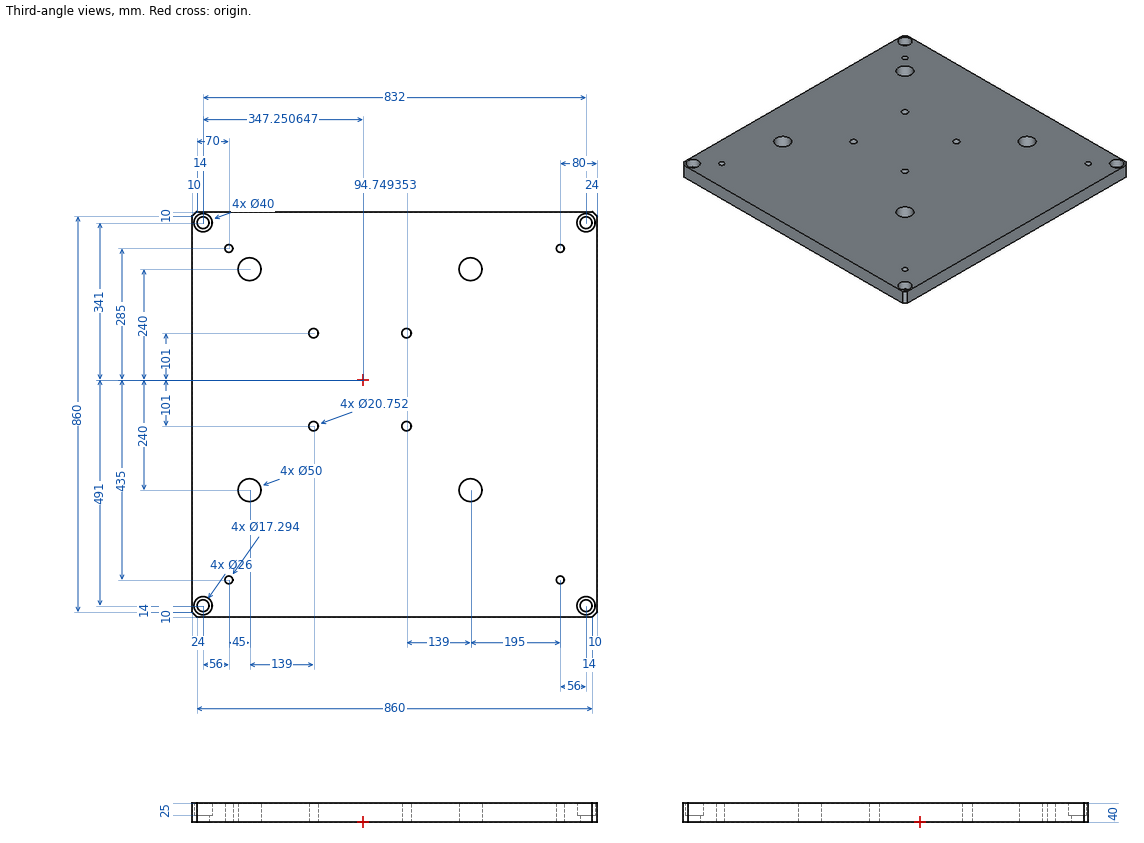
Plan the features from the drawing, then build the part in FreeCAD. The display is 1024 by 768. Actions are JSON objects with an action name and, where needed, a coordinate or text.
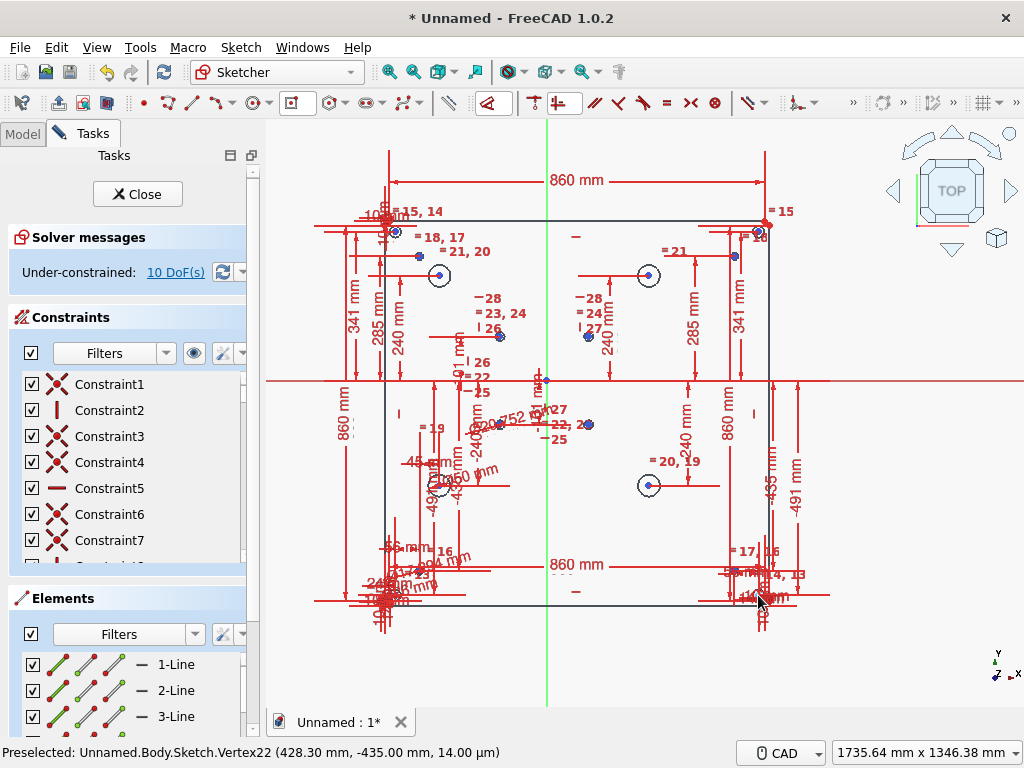
{"action": "scroll", "coordinate": [440, 276], "scroll_direction": "up", "scroll_amount": 4}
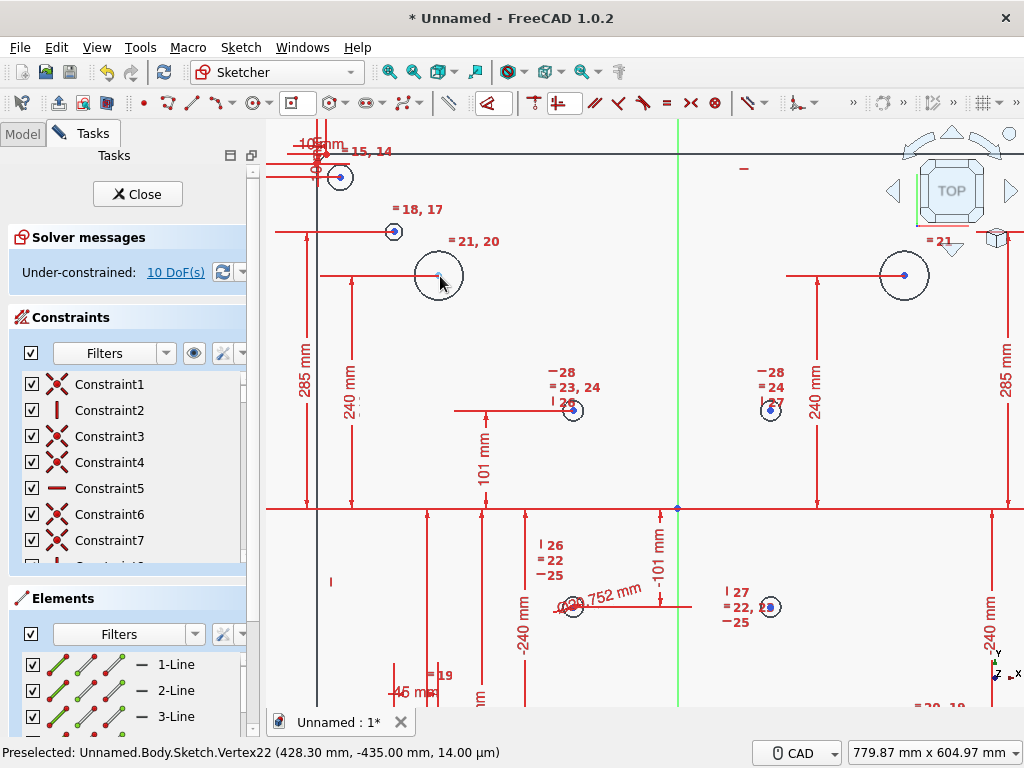
{"action": "left_click", "coordinate": [439, 276]}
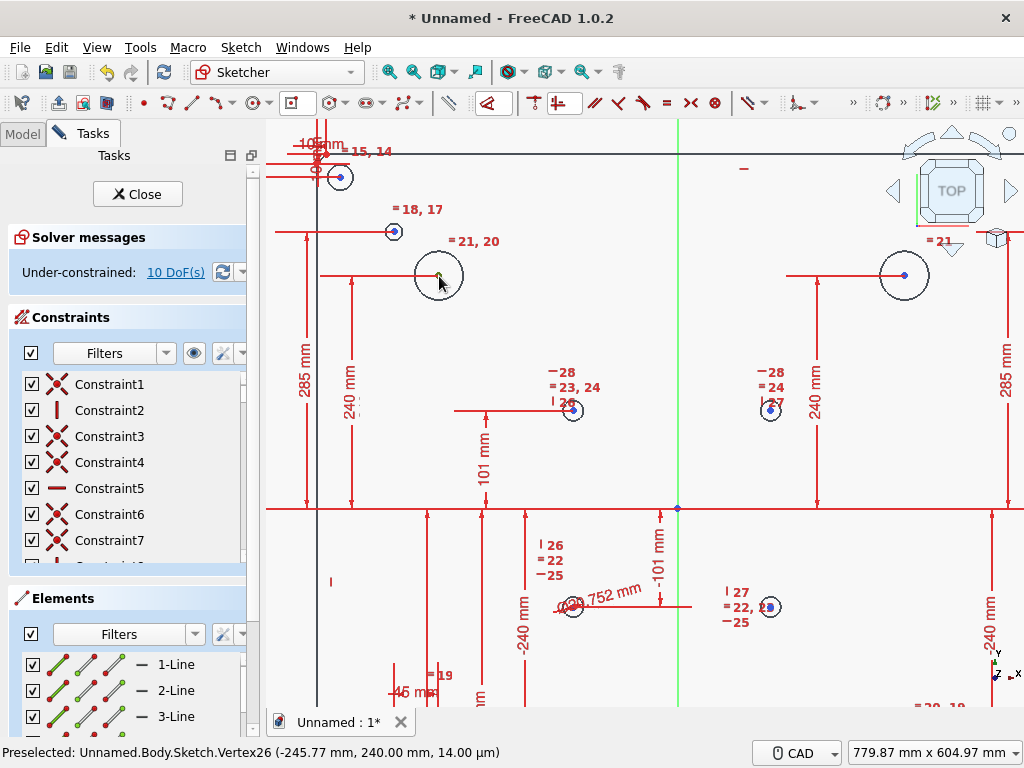
{"action": "left_click", "coordinate": [394, 232]}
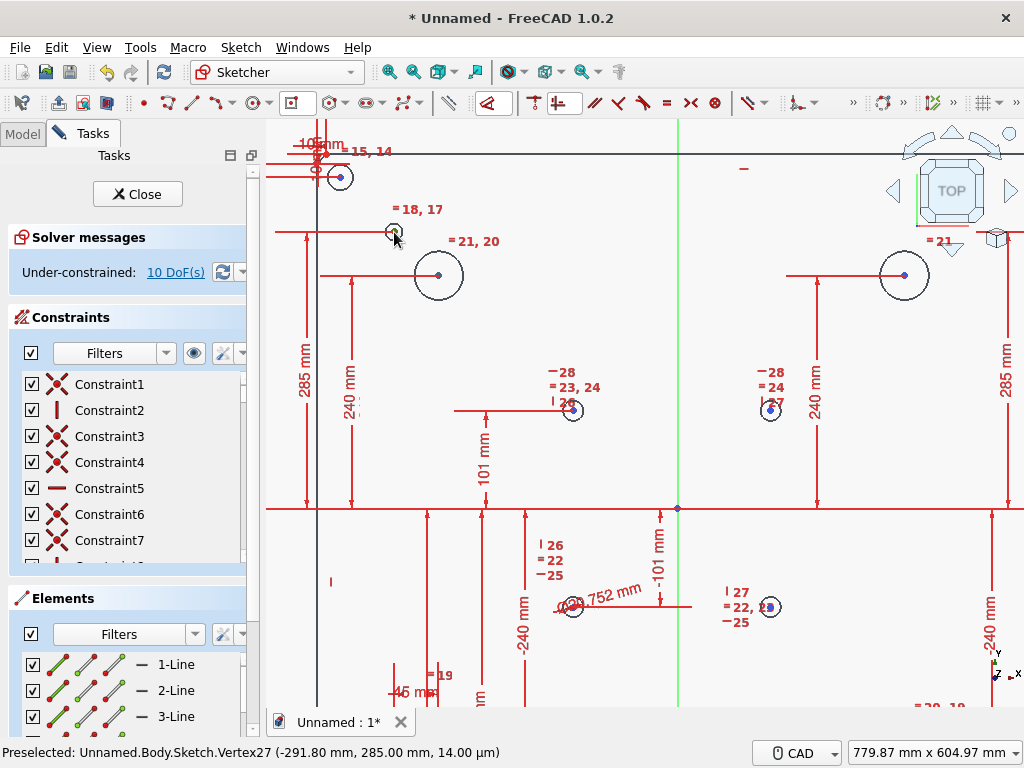
{"action": "key", "text": "l"}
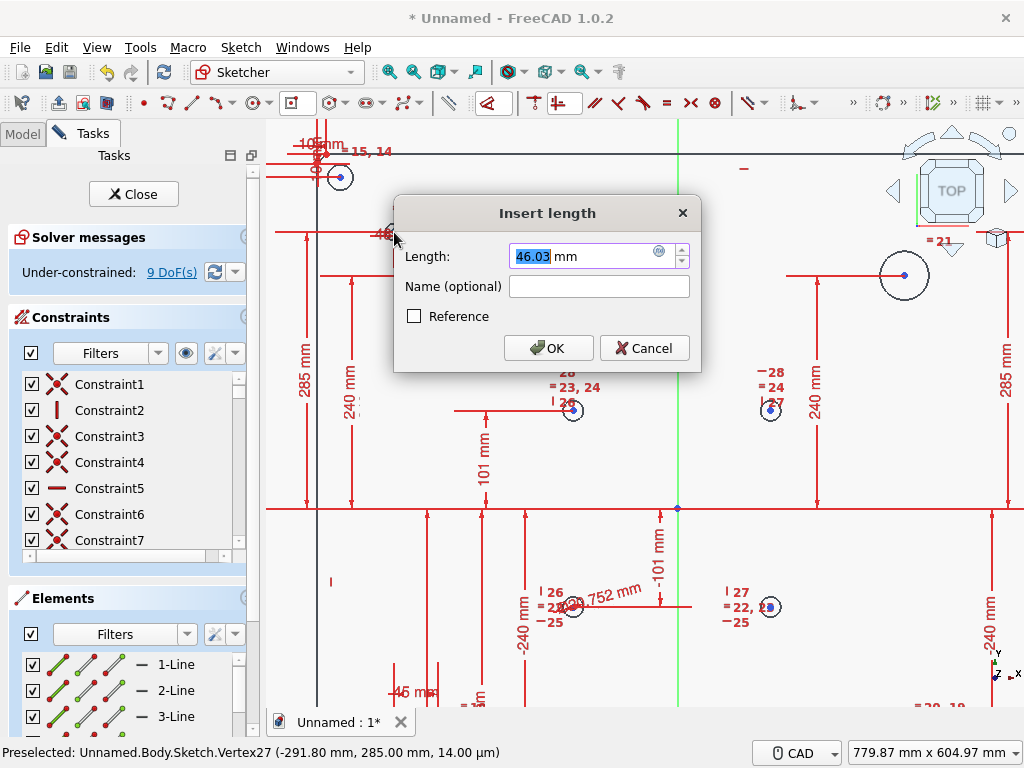
{"action": "type", "text": "45"}
{"action": "key", "text": "Return"}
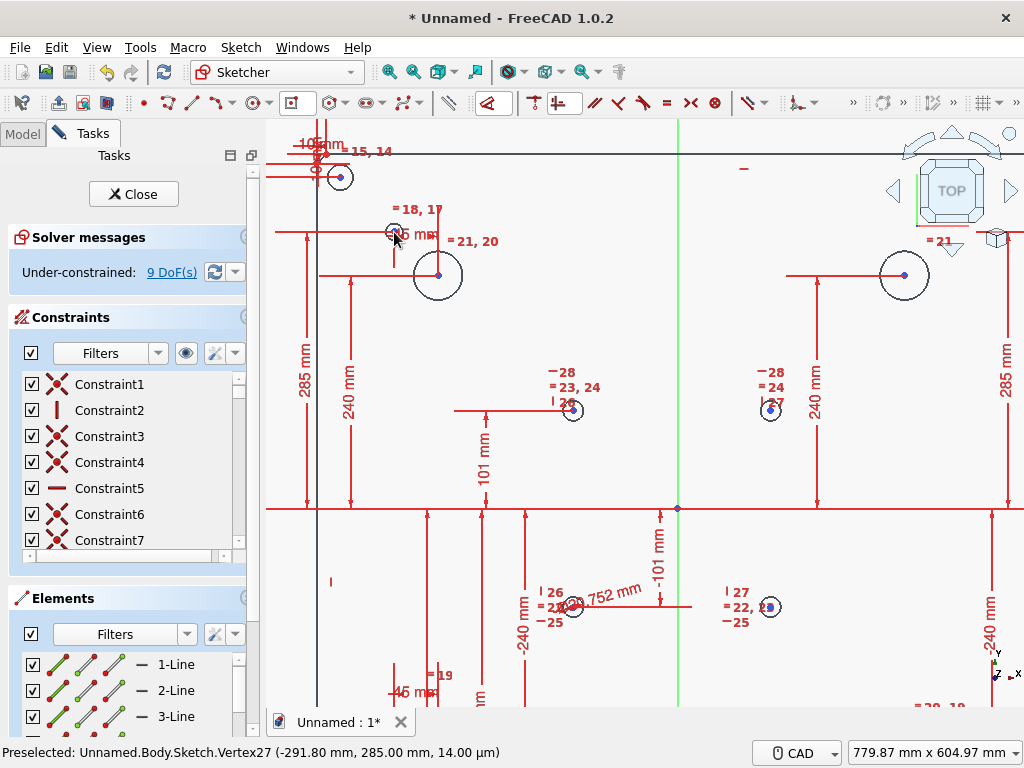
{"action": "left_click", "coordinate": [326, 154]}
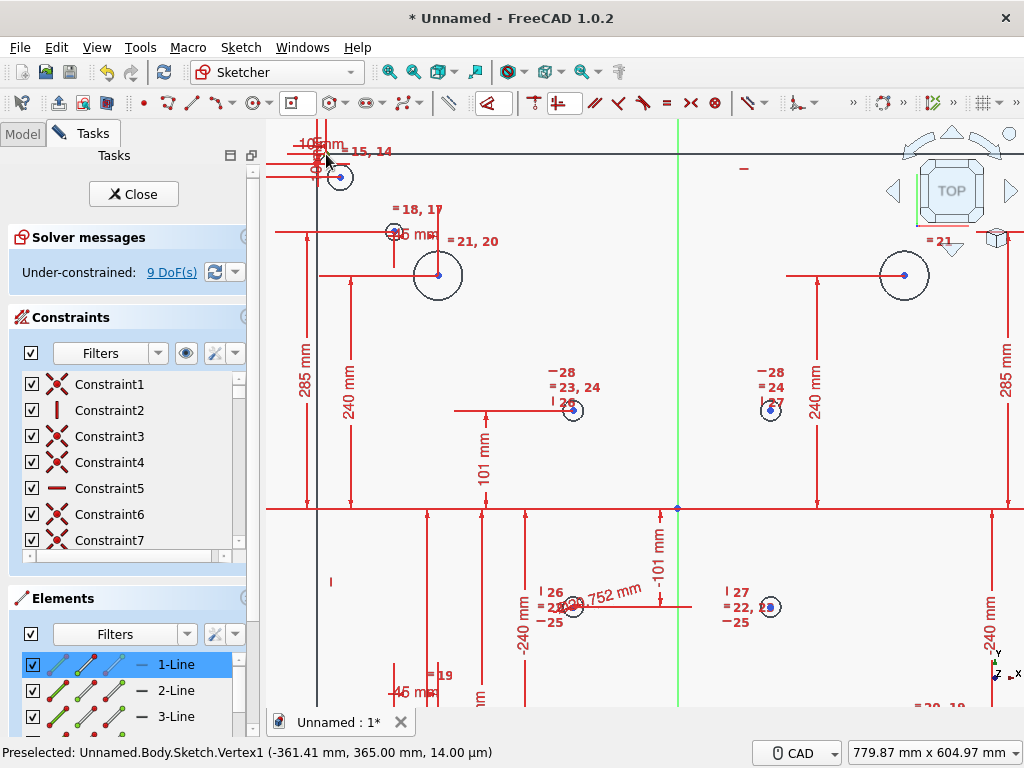
{"action": "left_click", "coordinate": [394, 232]}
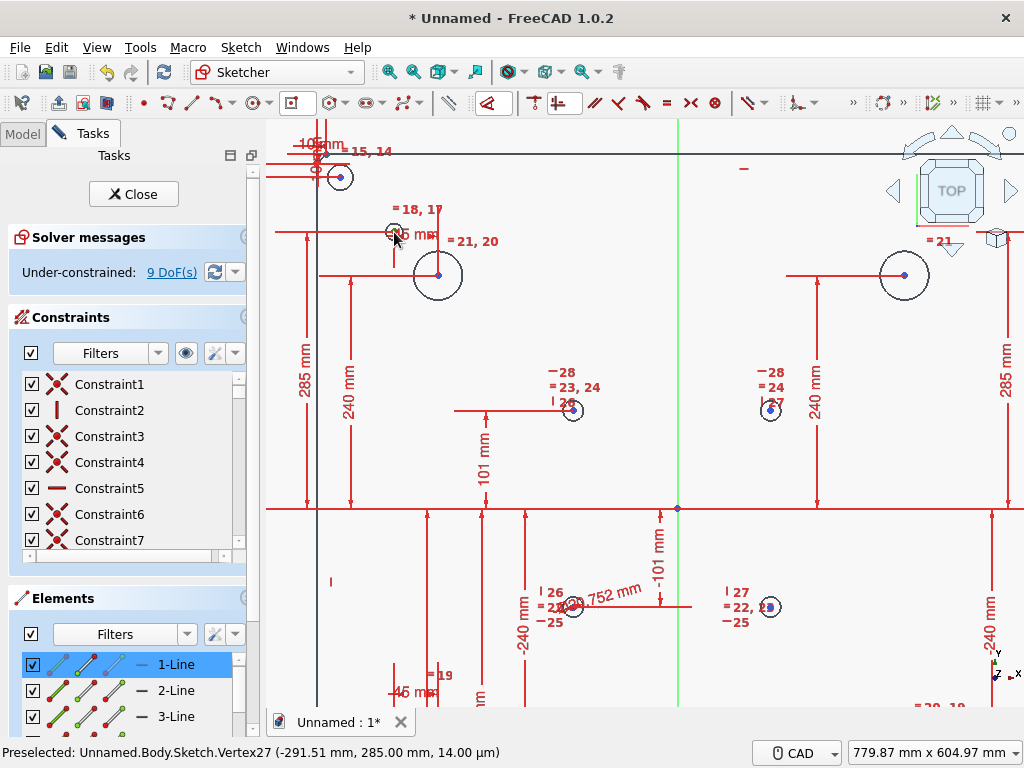
{"action": "key", "text": "l"}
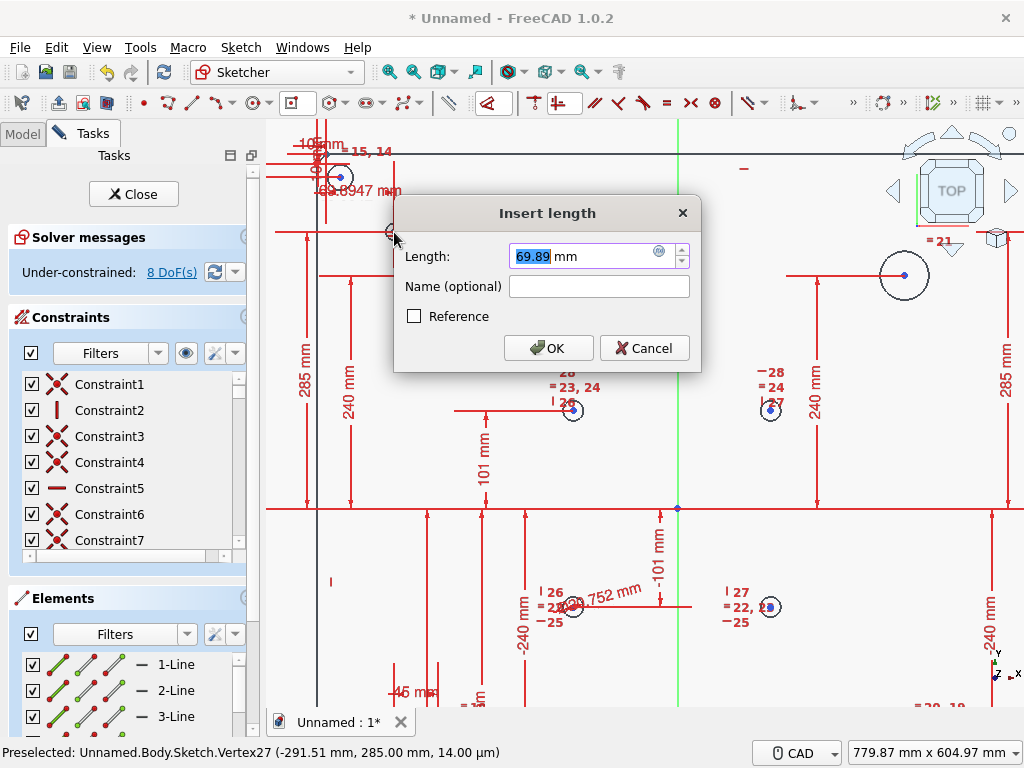
{"action": "type", "text": "70"}
{"action": "key", "text": "Return"}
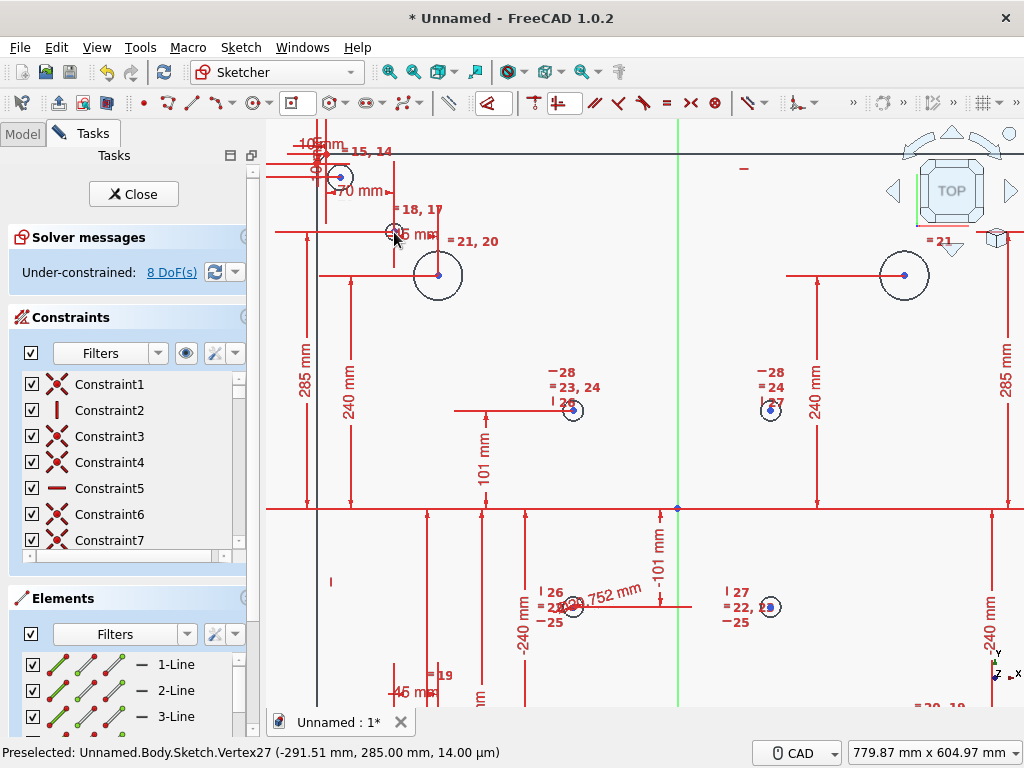
{"action": "scroll", "coordinate": [326, 154], "scroll_direction": "up", "scroll_amount": 6}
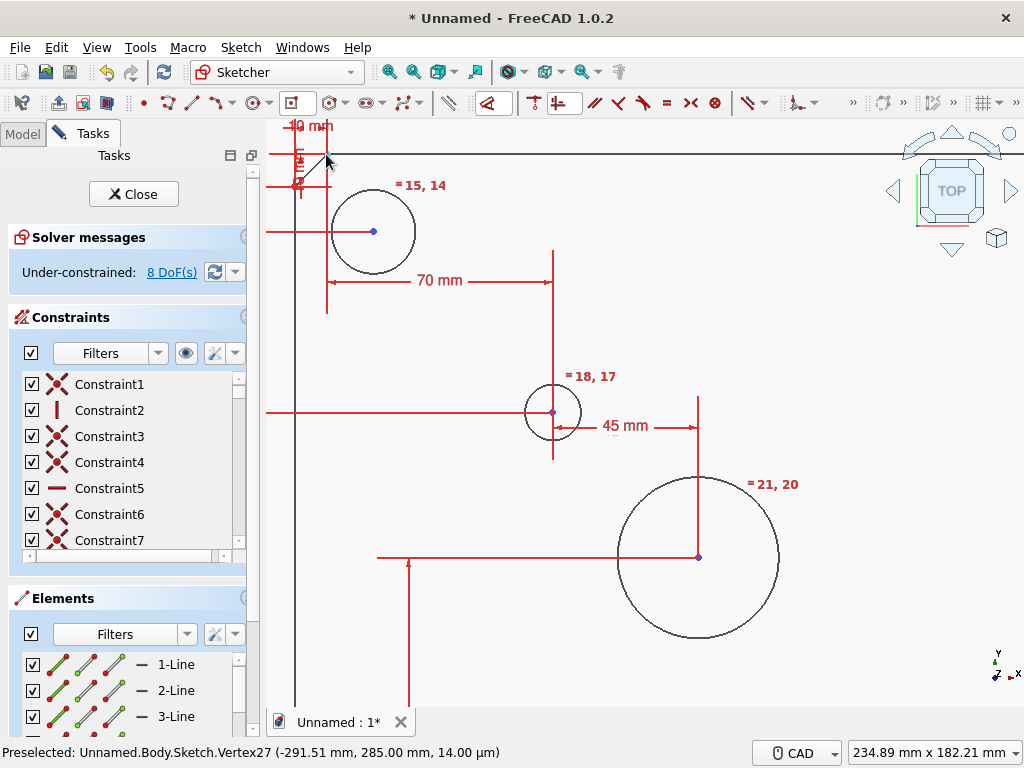
{"action": "left_click", "coordinate": [327, 154]}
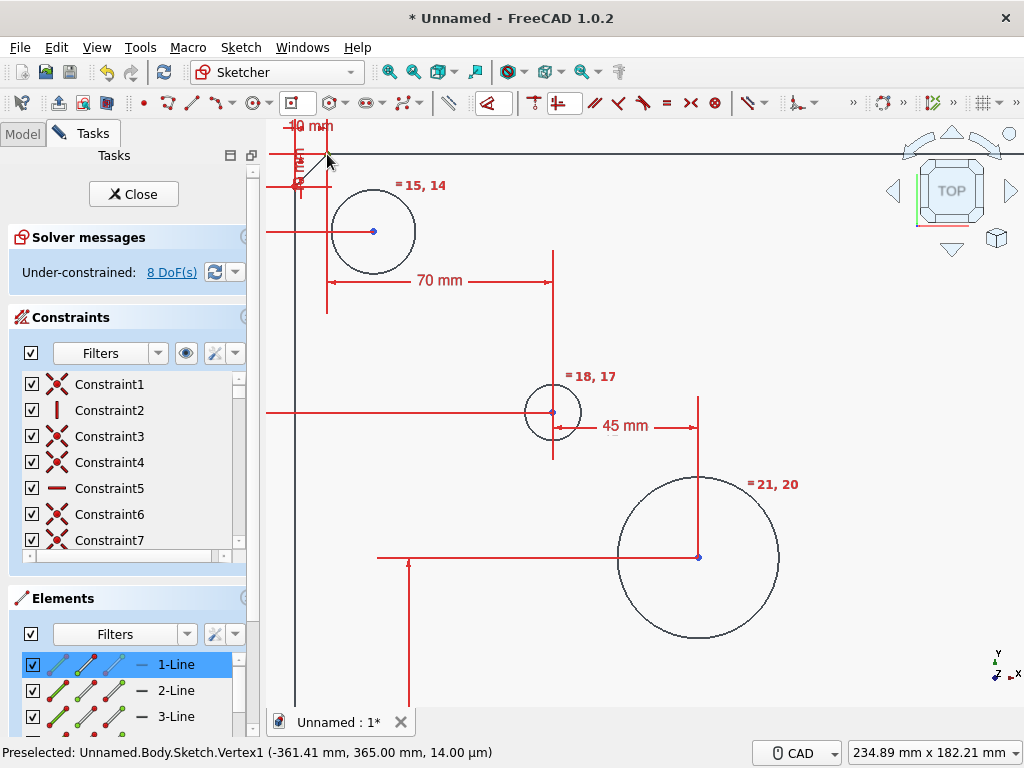
{"action": "left_click", "coordinate": [374, 232]}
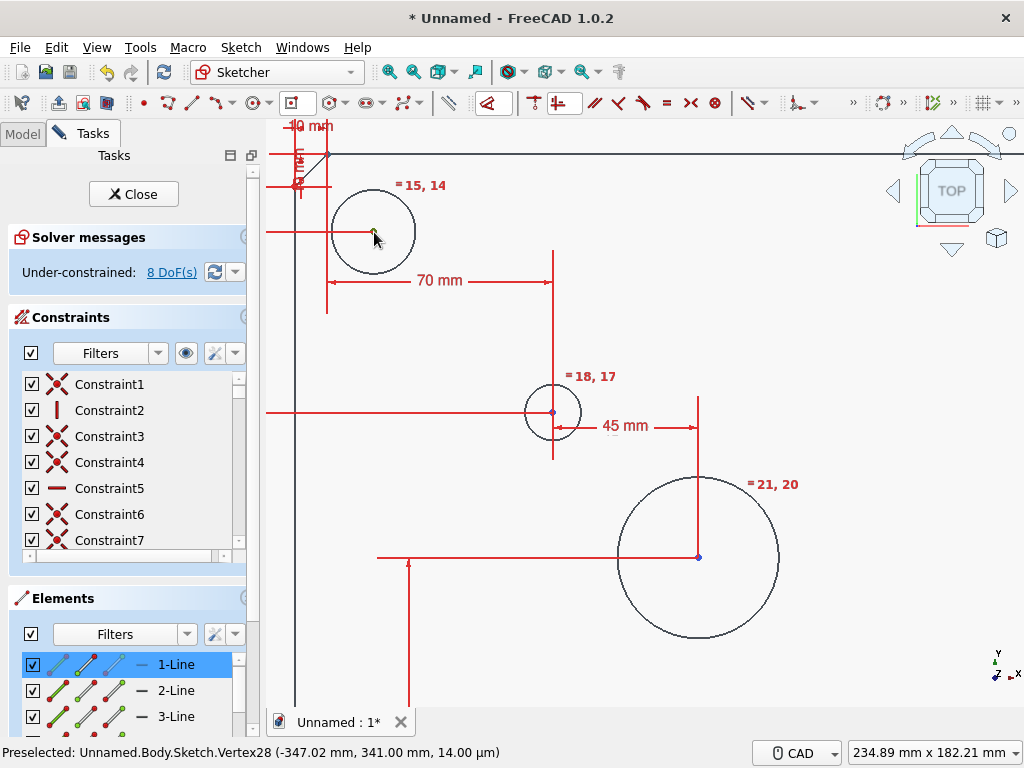
{"action": "key", "text": "l"}